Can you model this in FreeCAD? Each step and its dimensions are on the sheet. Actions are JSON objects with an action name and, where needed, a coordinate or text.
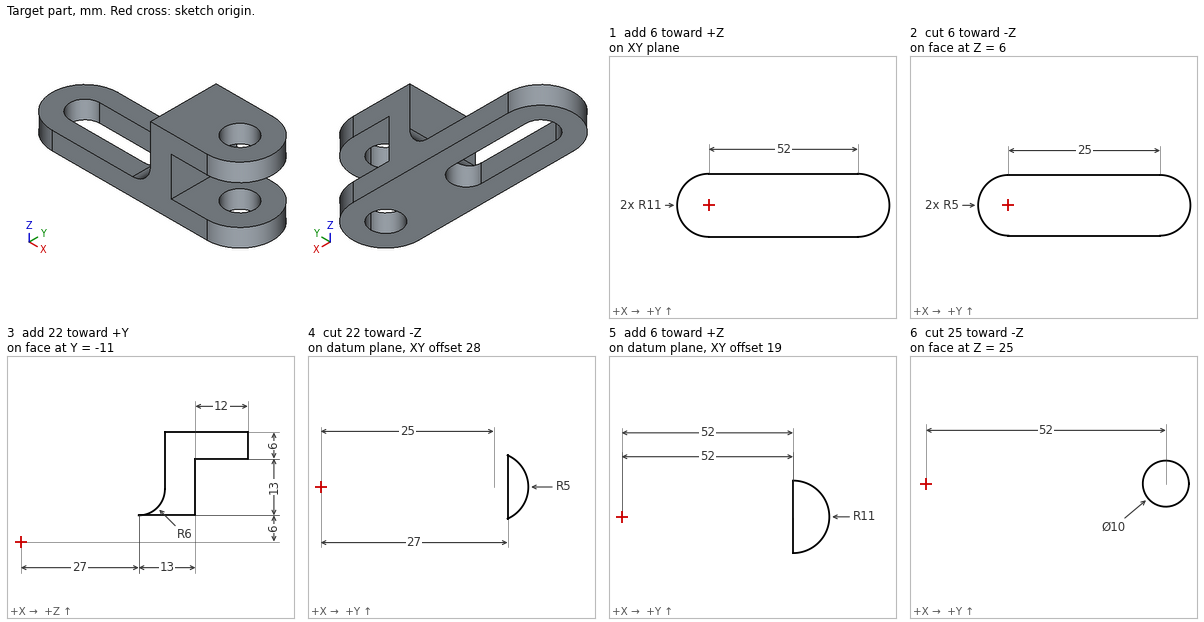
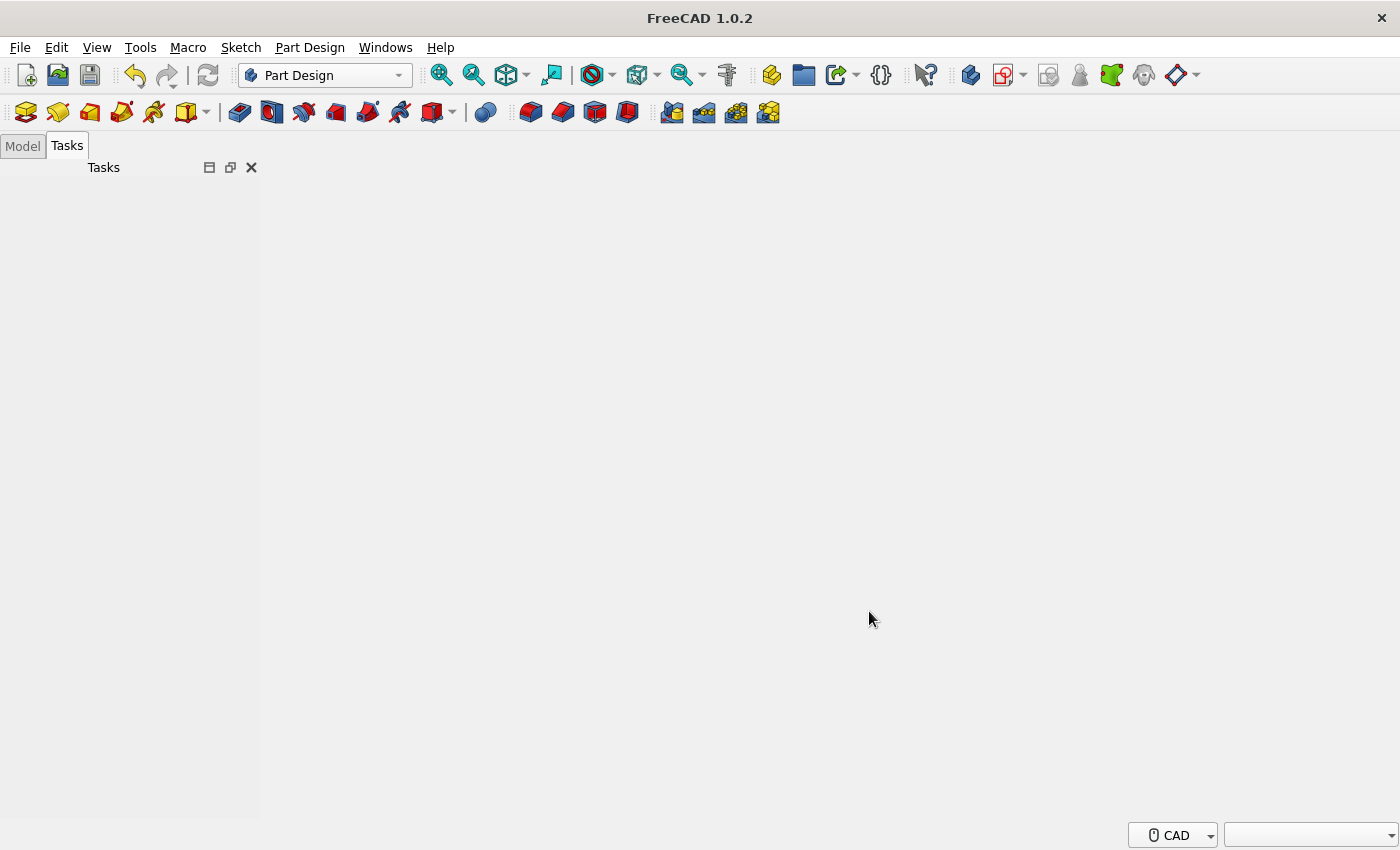
{"action": "left_click", "coordinate": [26, 76]}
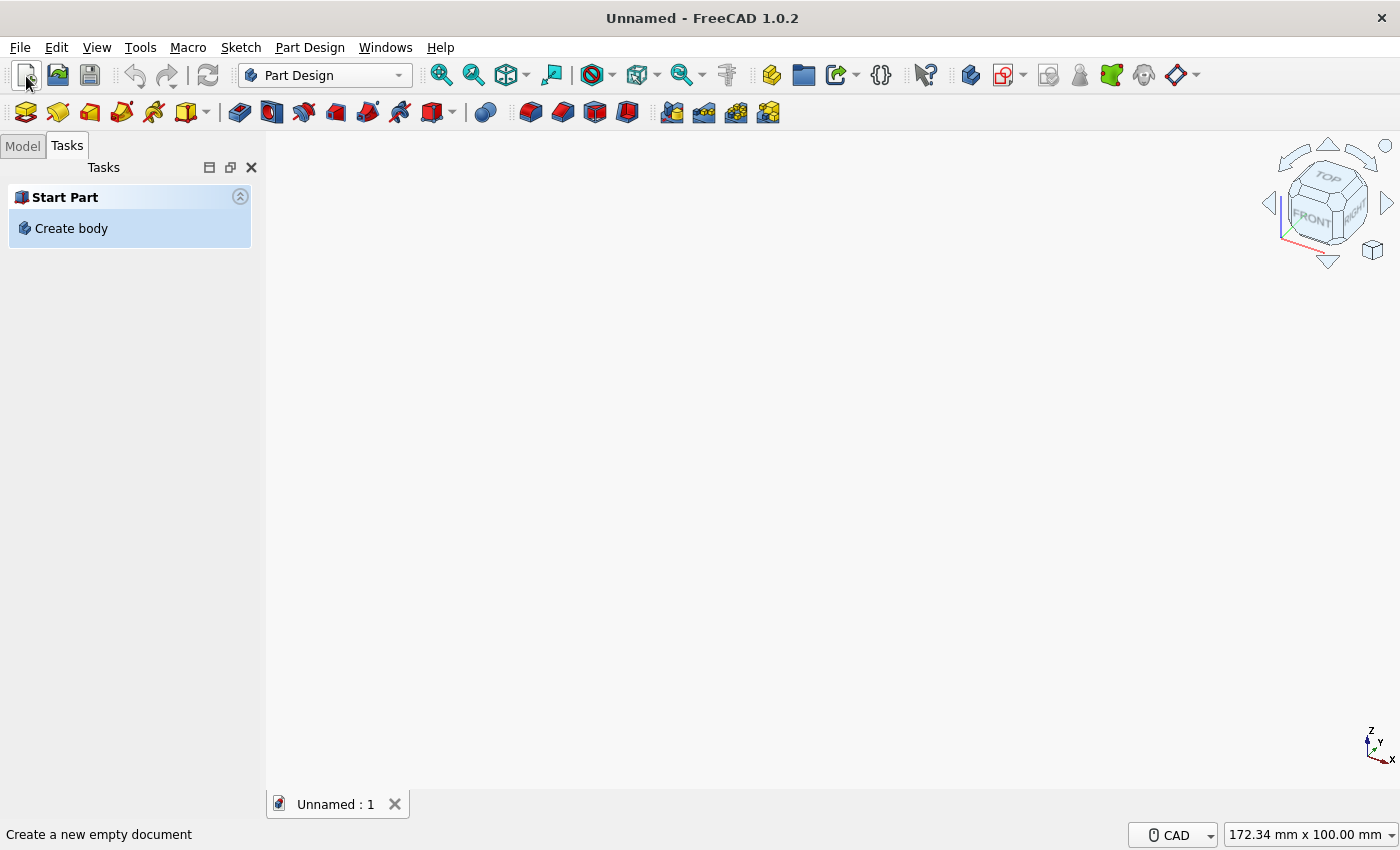
{"action": "left_click", "coordinate": [1004, 76]}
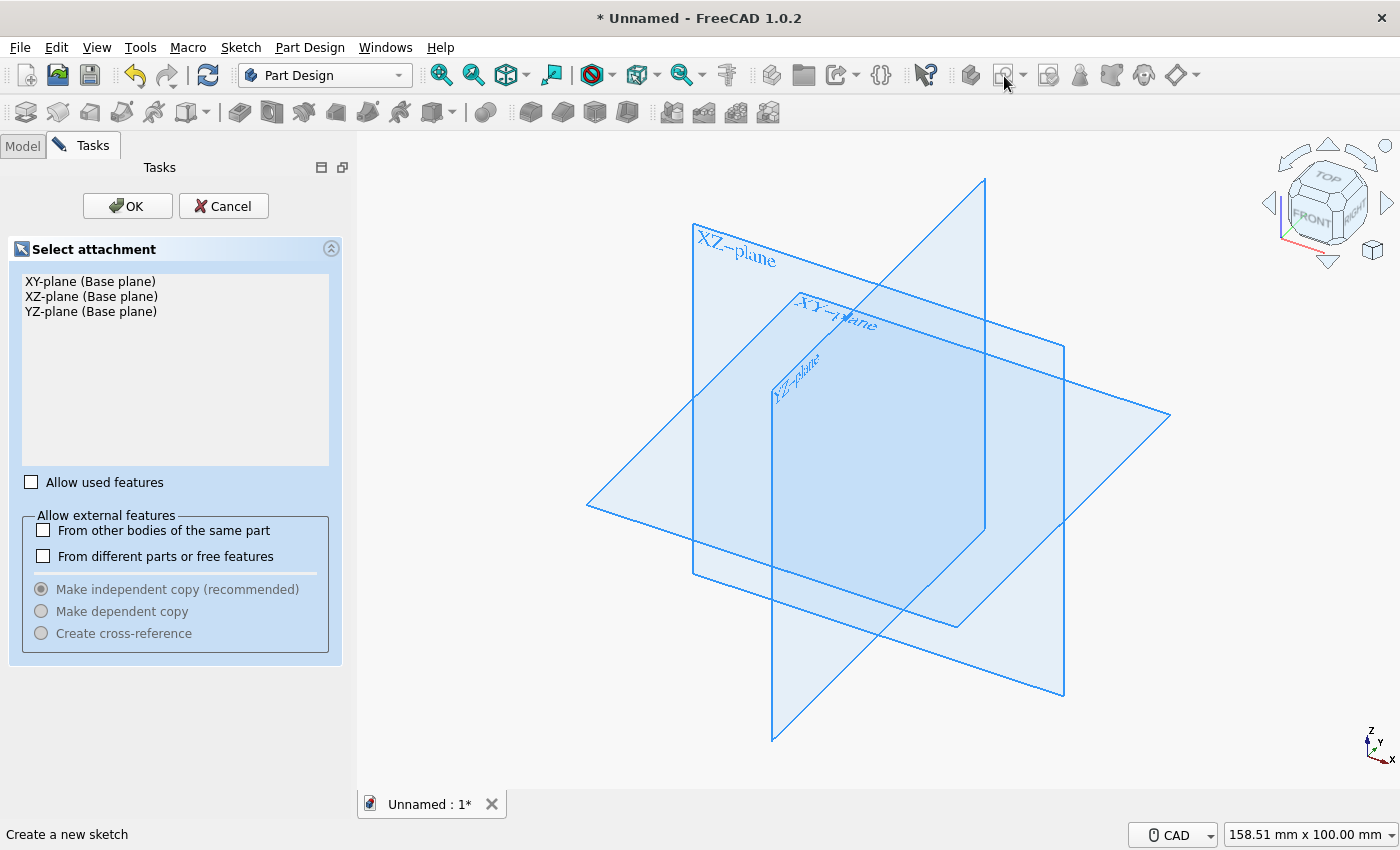
{"action": "left_click", "coordinate": [82, 282]}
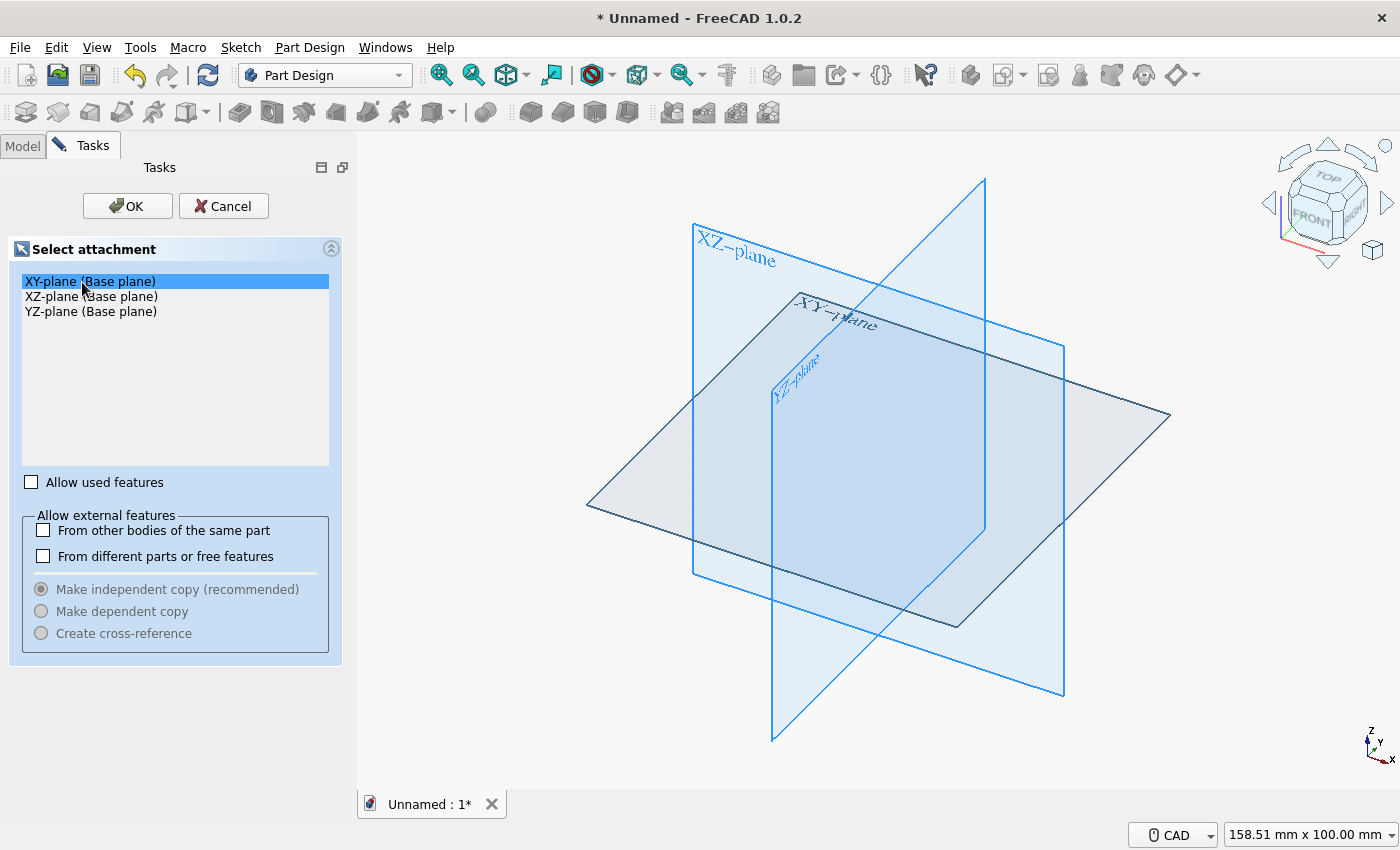
{"action": "left_click", "coordinate": [128, 206]}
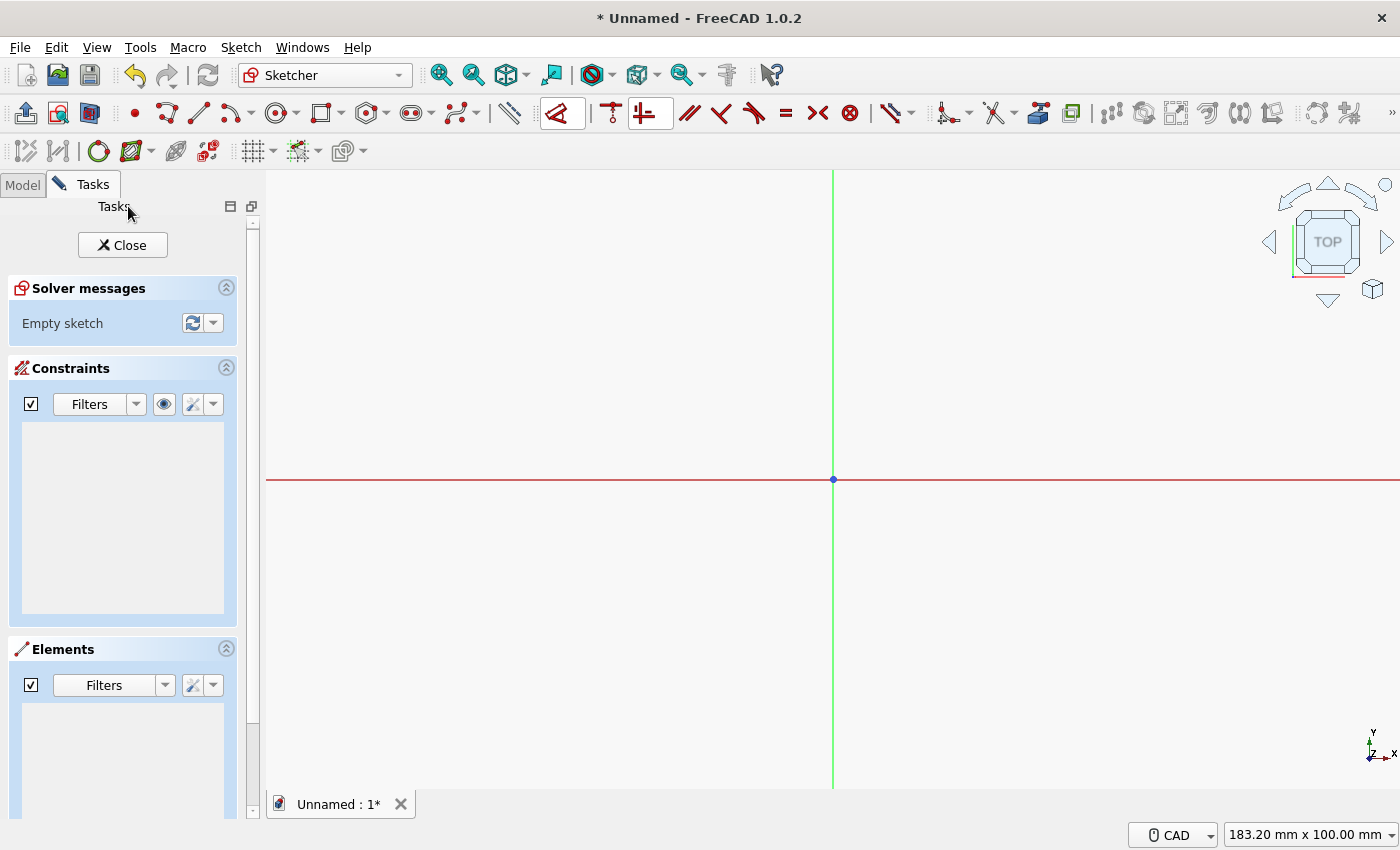
{"action": "scroll", "coordinate": [294, 480], "scroll_direction": "down", "scroll_amount": 1}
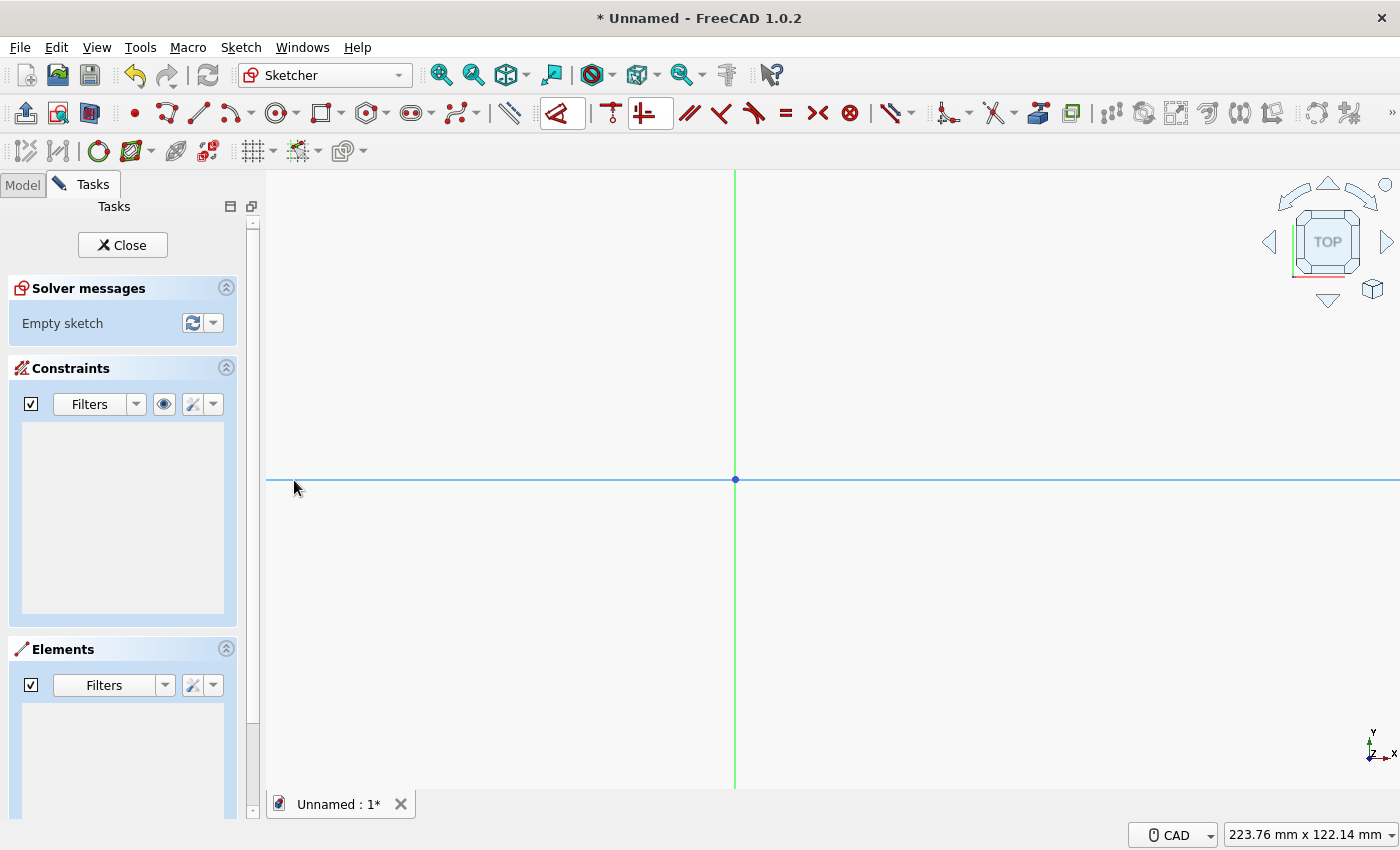
{"action": "scroll", "coordinate": [992, 480], "scroll_direction": "up", "scroll_amount": 3}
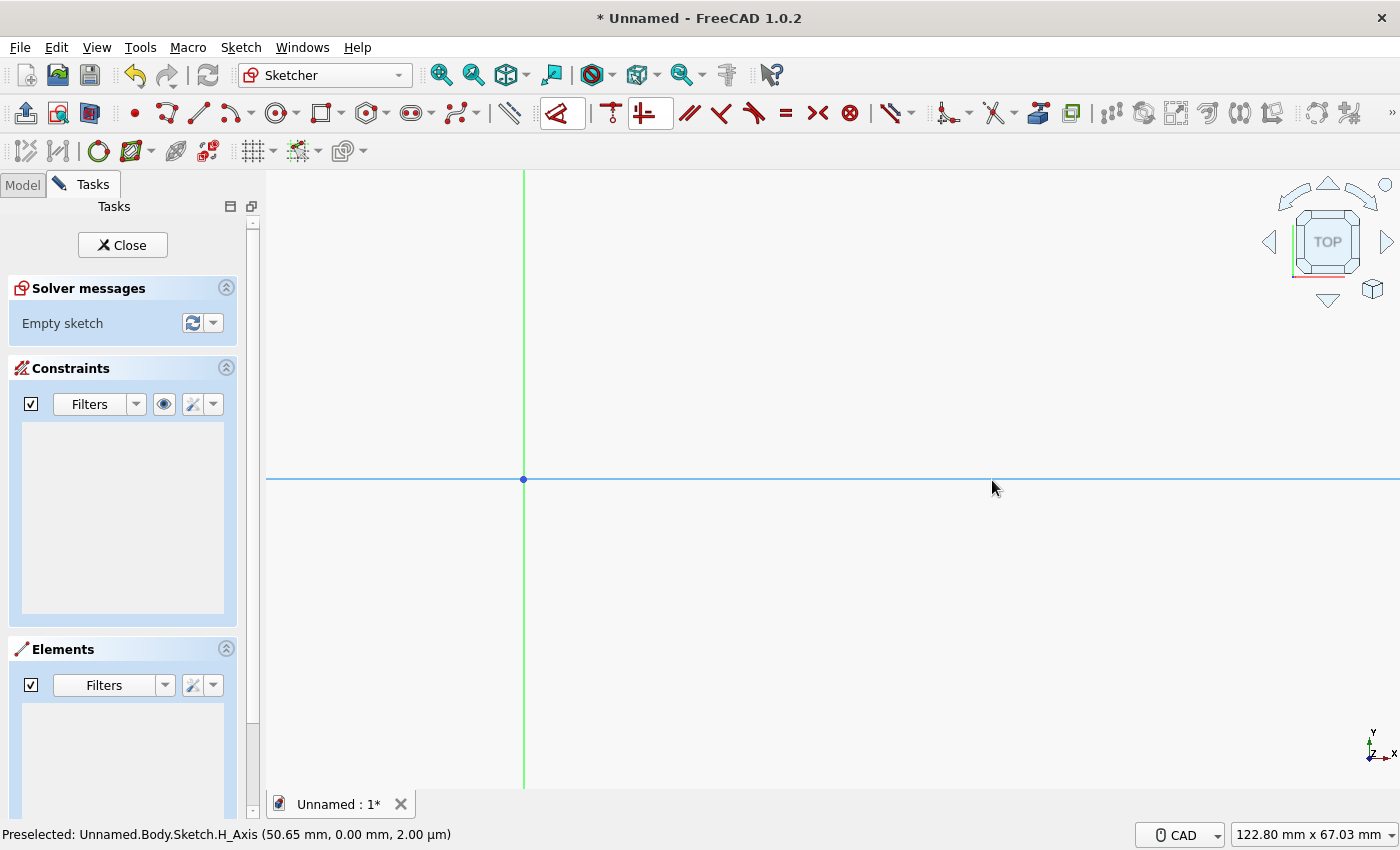
{"action": "left_click", "coordinate": [412, 114]}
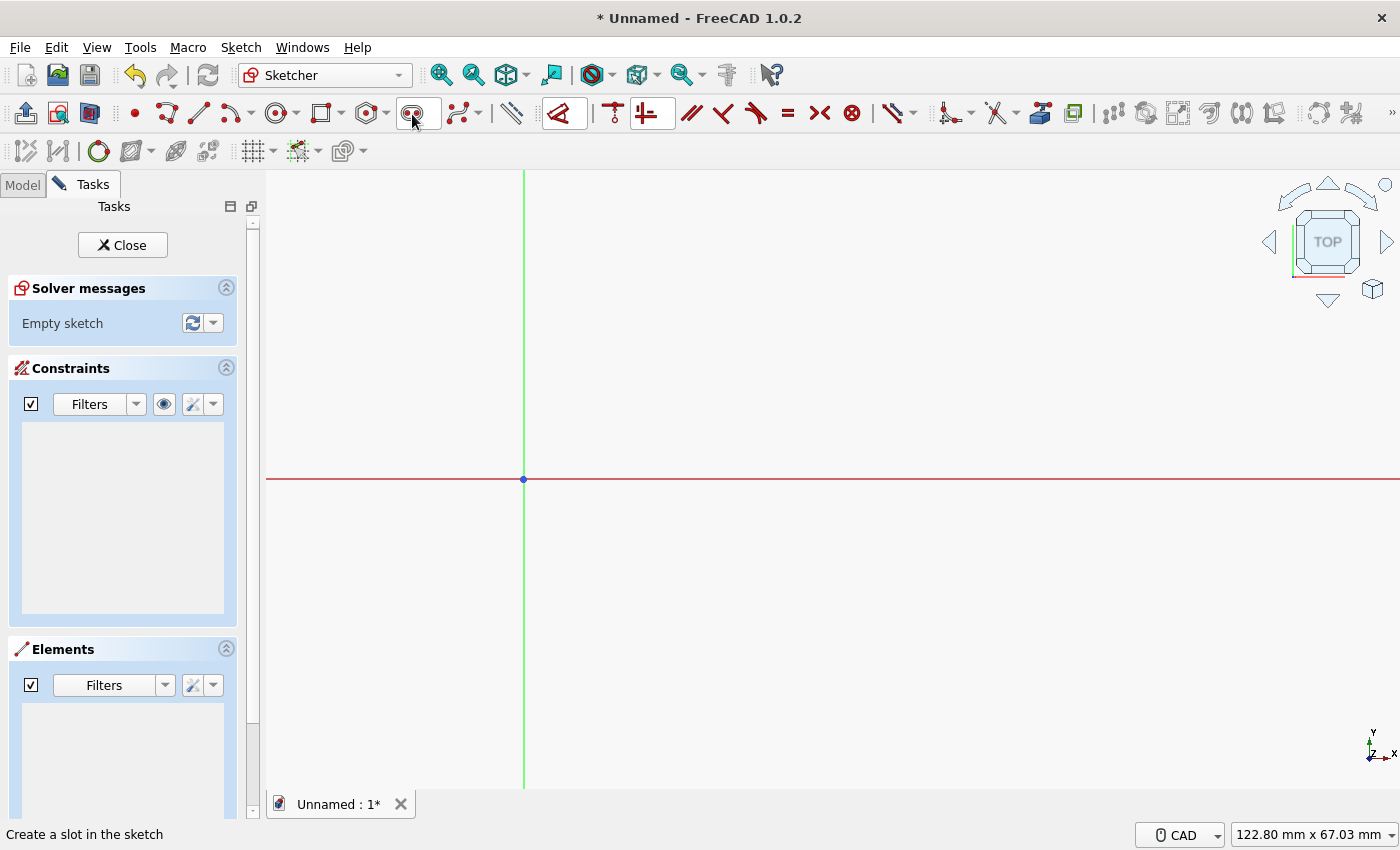
{"action": "left_click", "coordinate": [524, 479]}